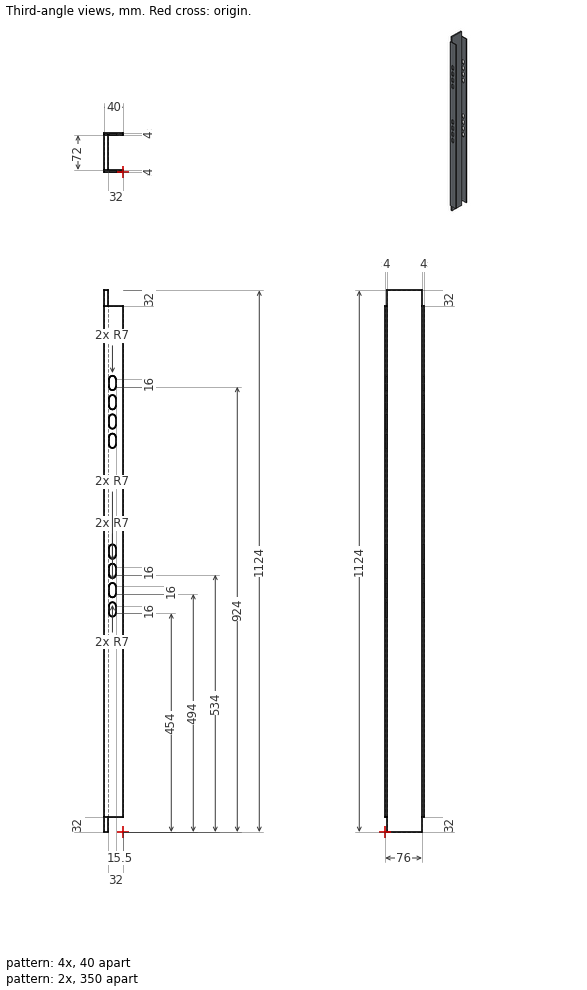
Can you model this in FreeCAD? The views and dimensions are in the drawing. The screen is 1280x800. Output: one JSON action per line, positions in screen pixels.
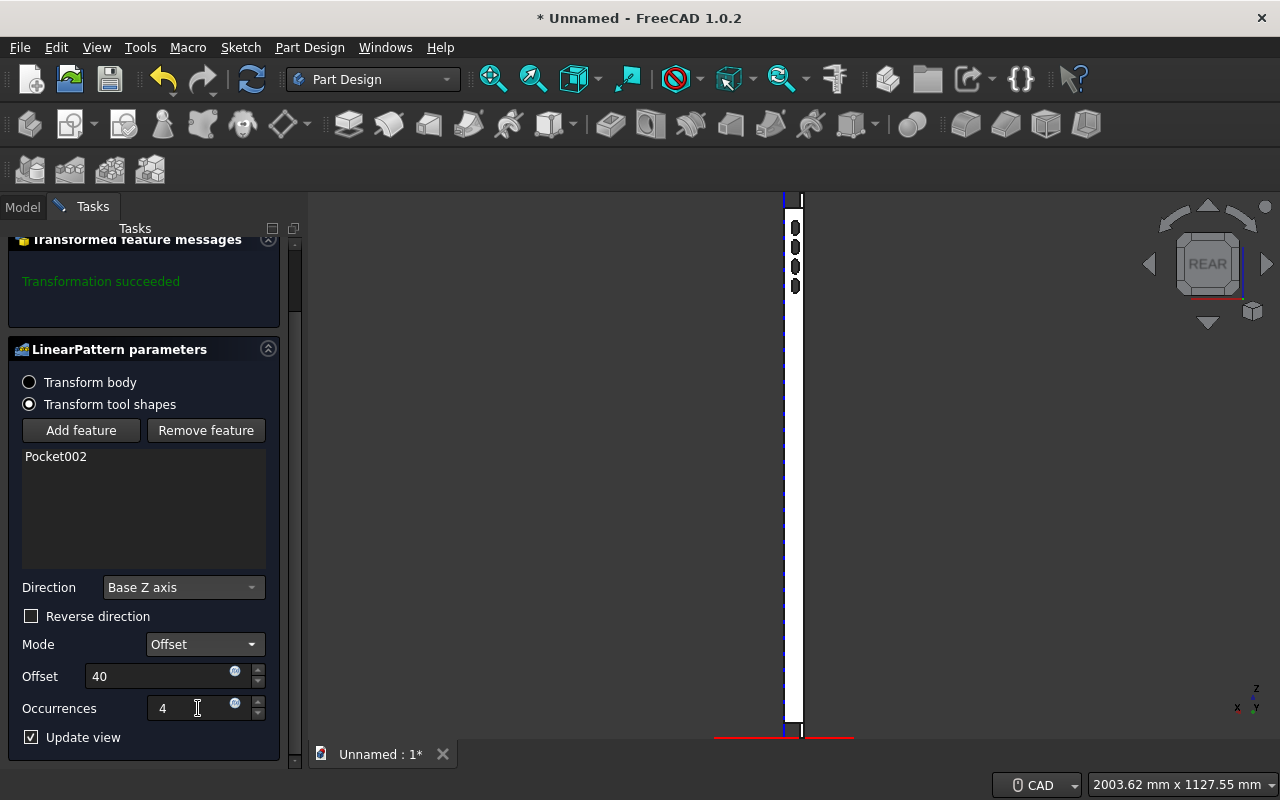
{"action": "left_click", "coordinate": [30, 616]}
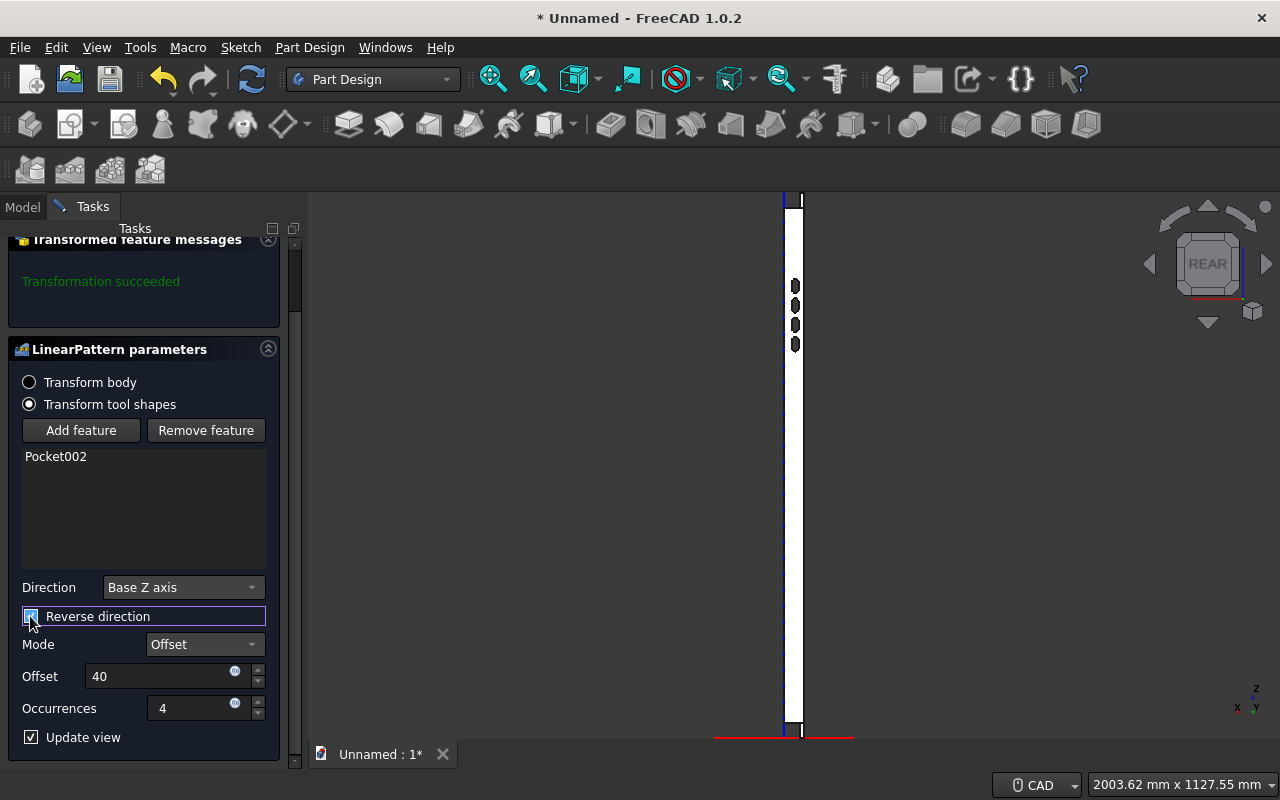
{"action": "scroll", "coordinate": [295, 503], "scroll_direction": "up", "scroll_amount": 2}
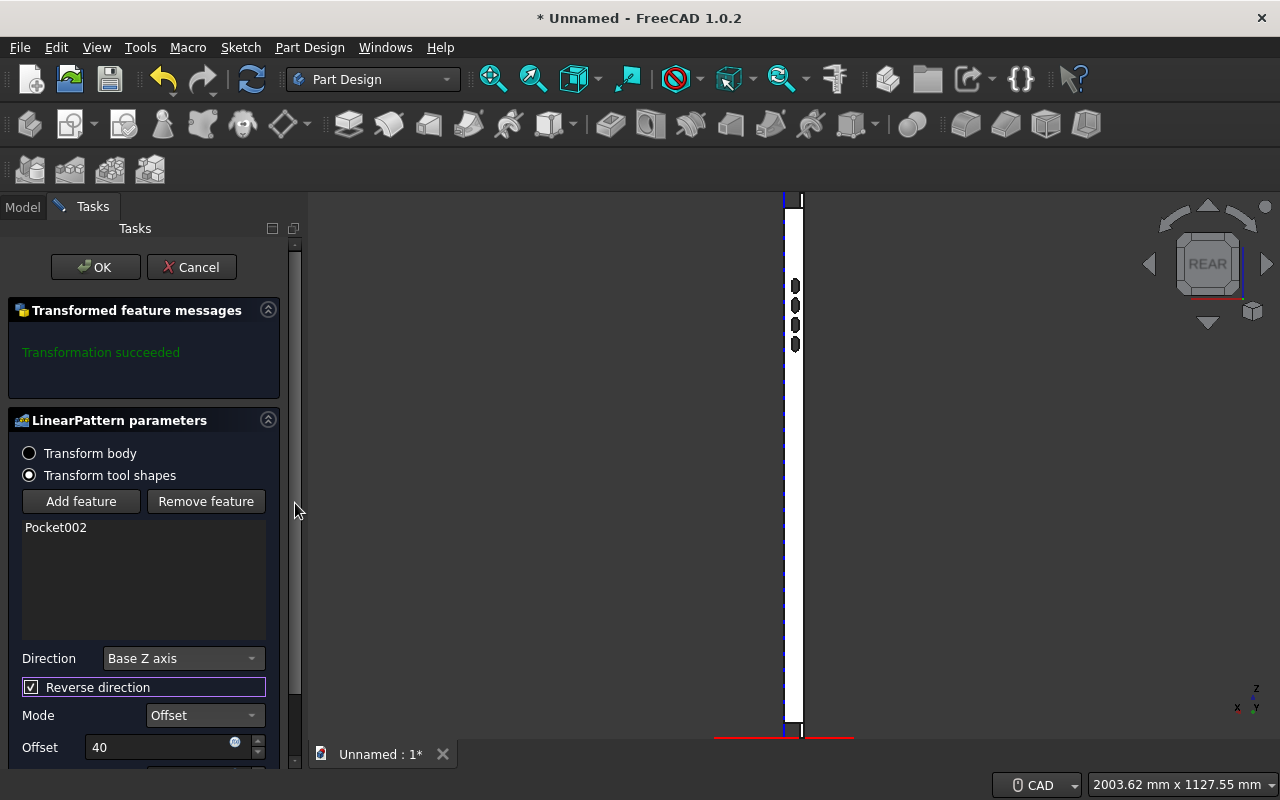
{"action": "left_click", "coordinate": [96, 267]}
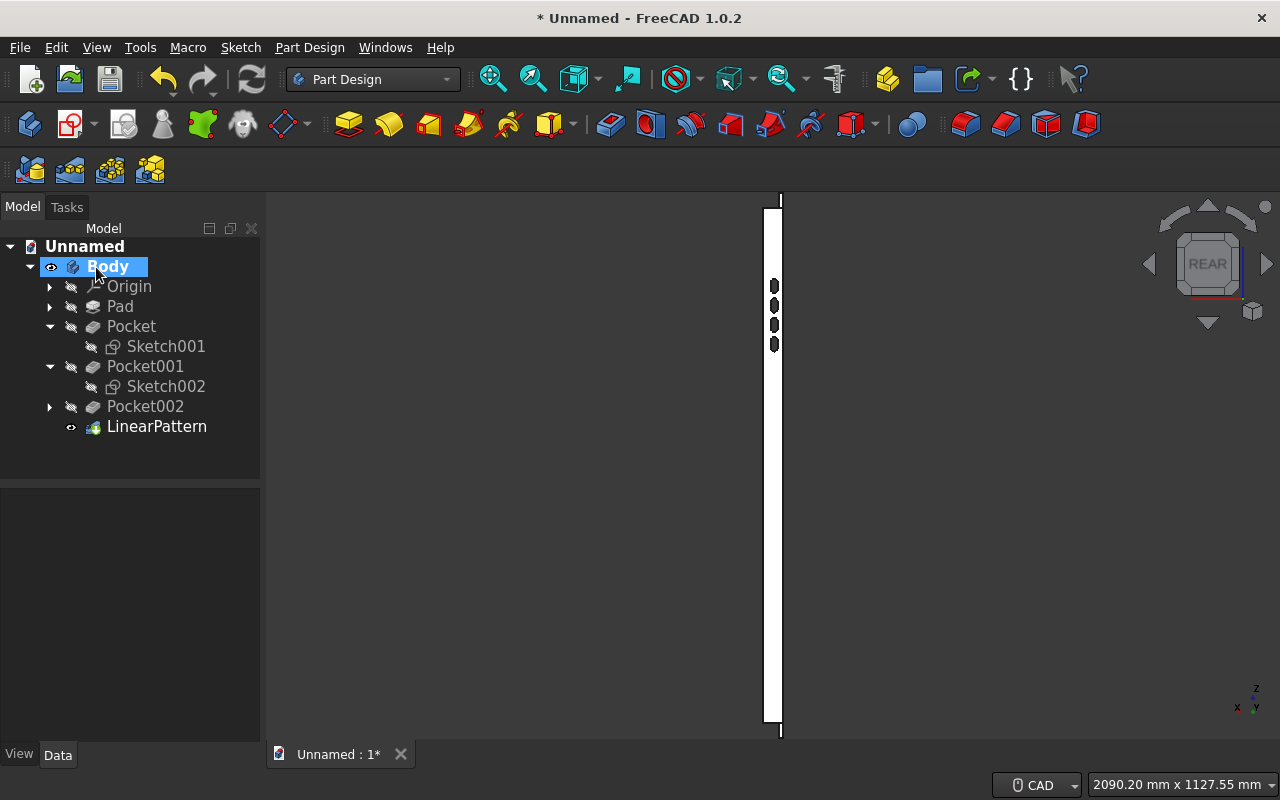
{"action": "left_click", "coordinate": [116, 407]}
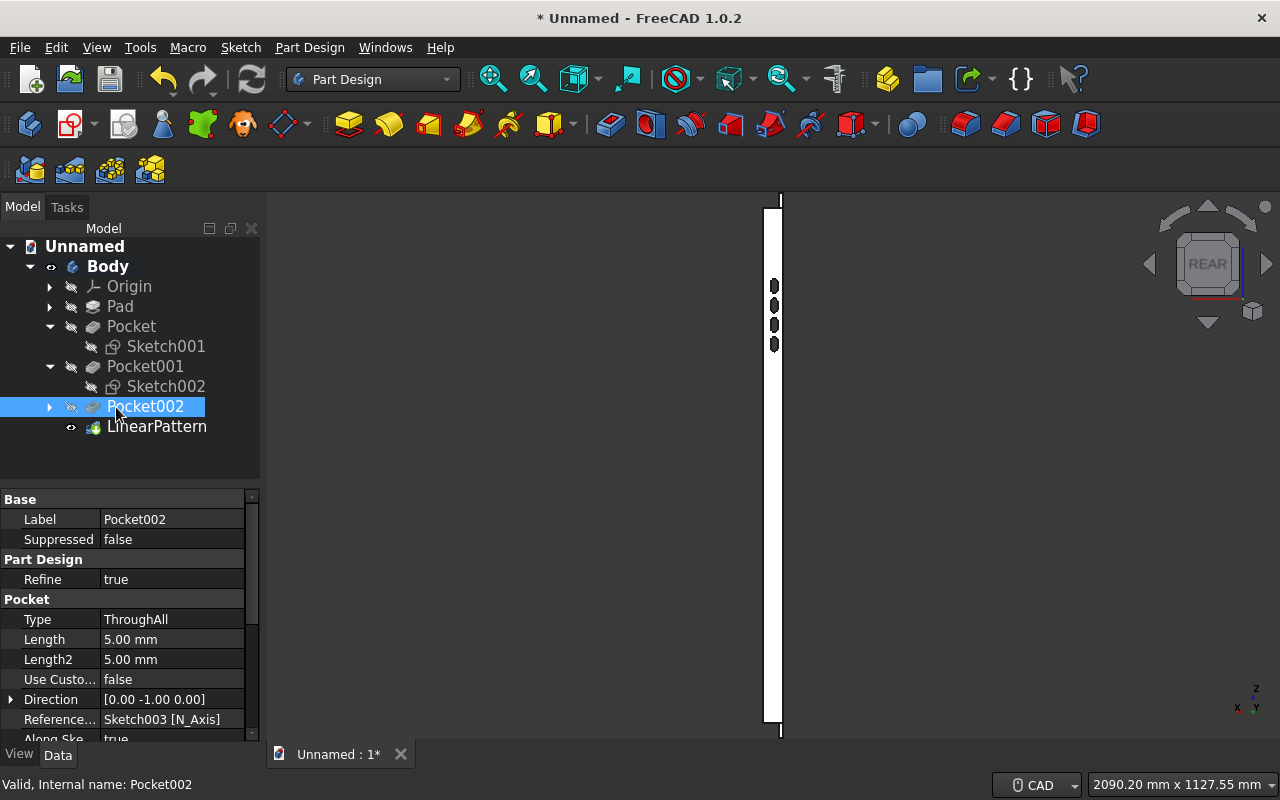
{"action": "left_click", "coordinate": [70, 170]}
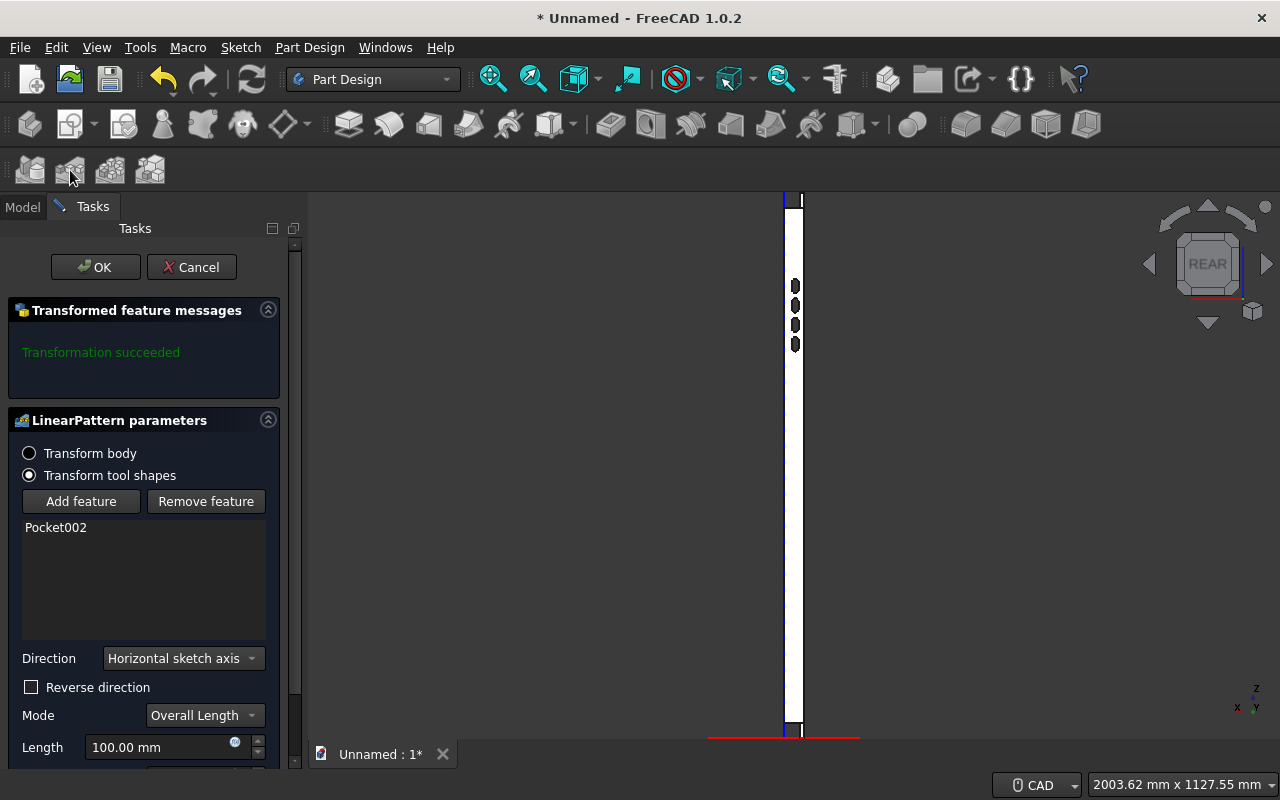
{"action": "left_click", "coordinate": [184, 658]}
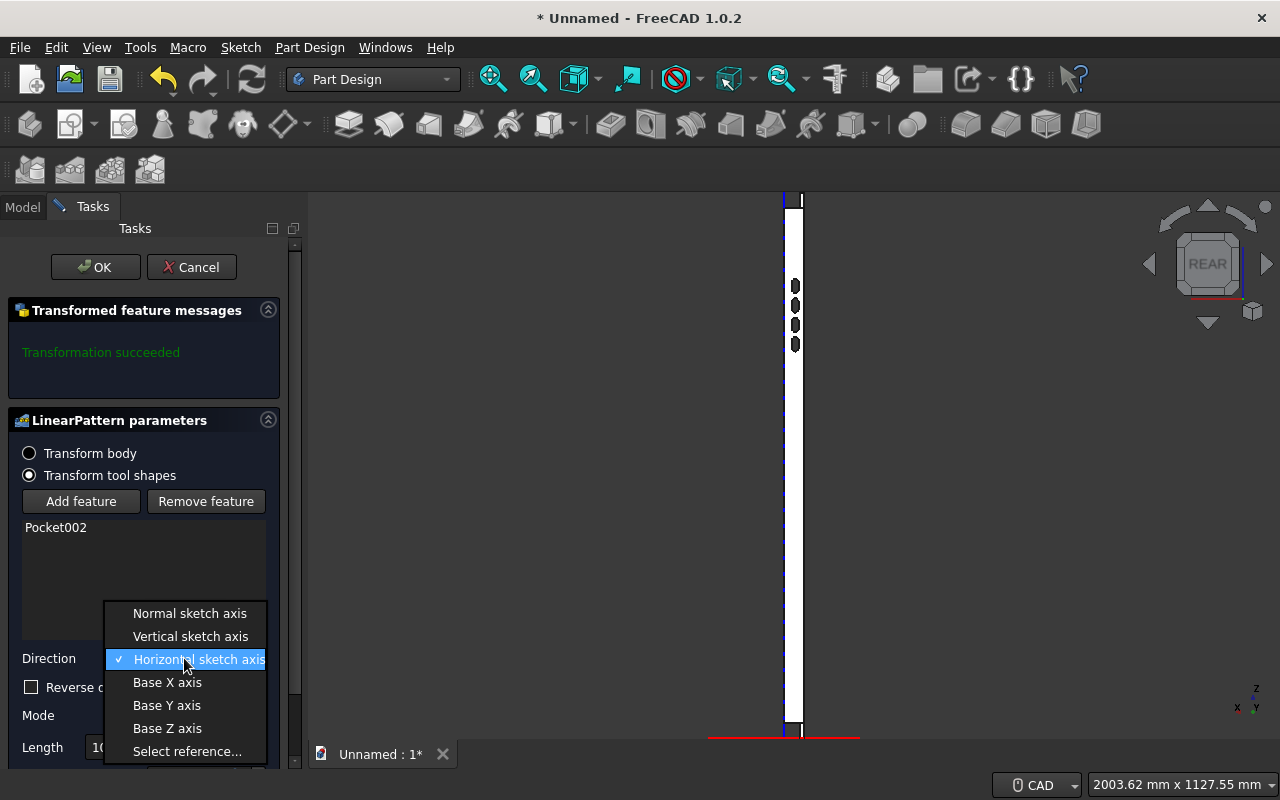
{"action": "left_click", "coordinate": [184, 728]}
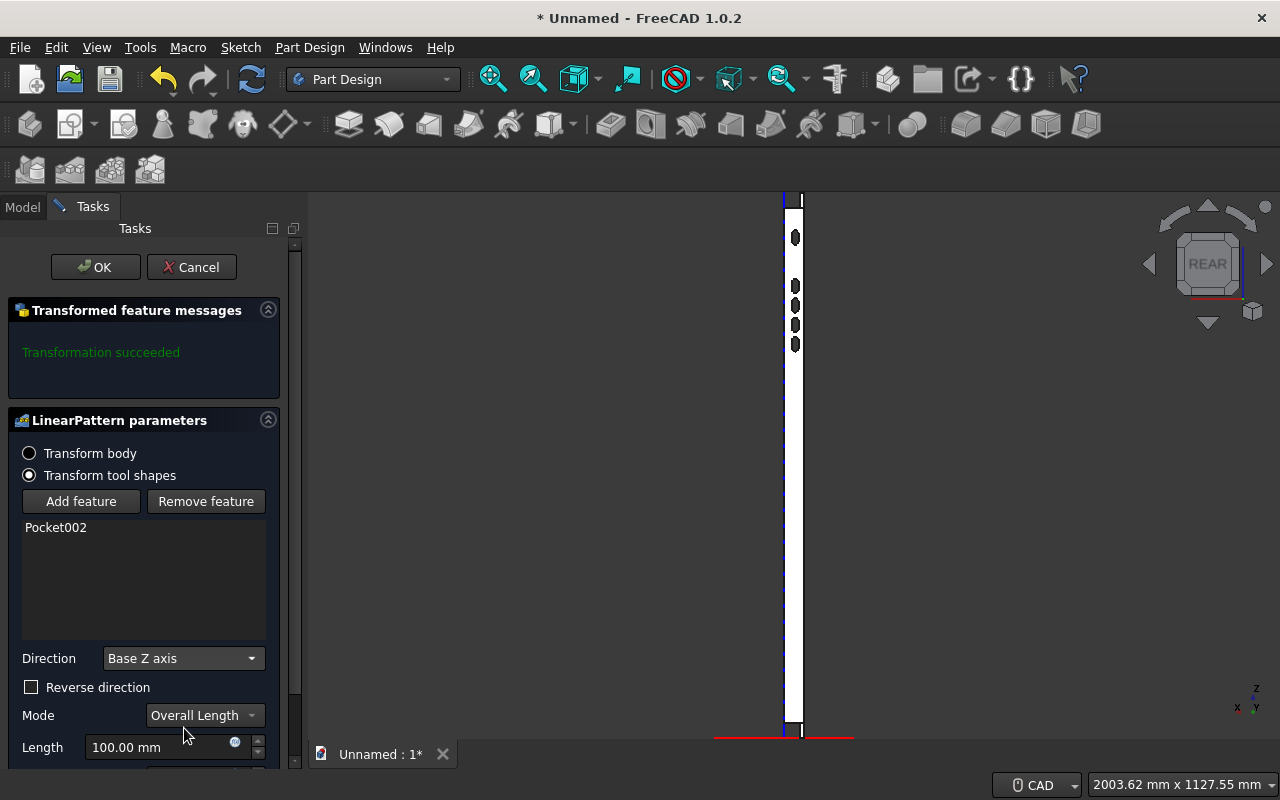
{"action": "left_click", "coordinate": [206, 716]}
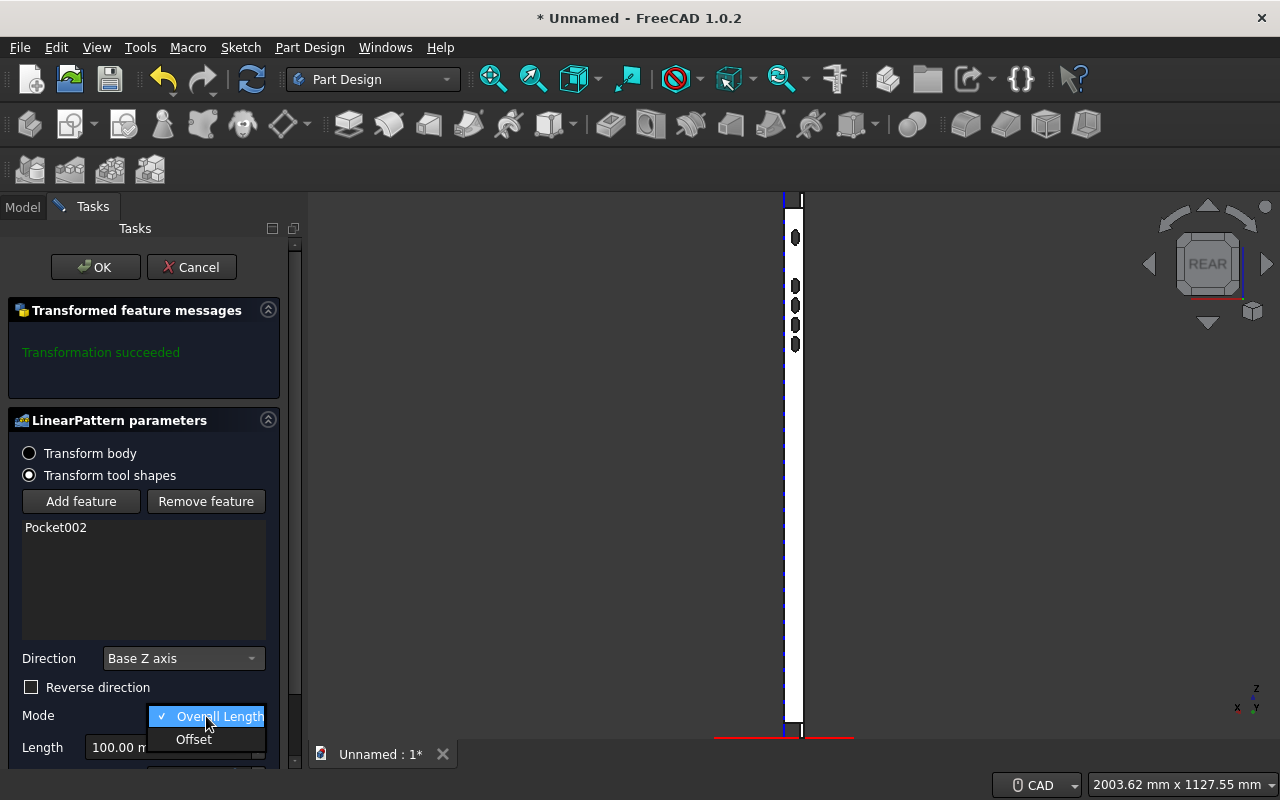
{"action": "left_click", "coordinate": [206, 740]}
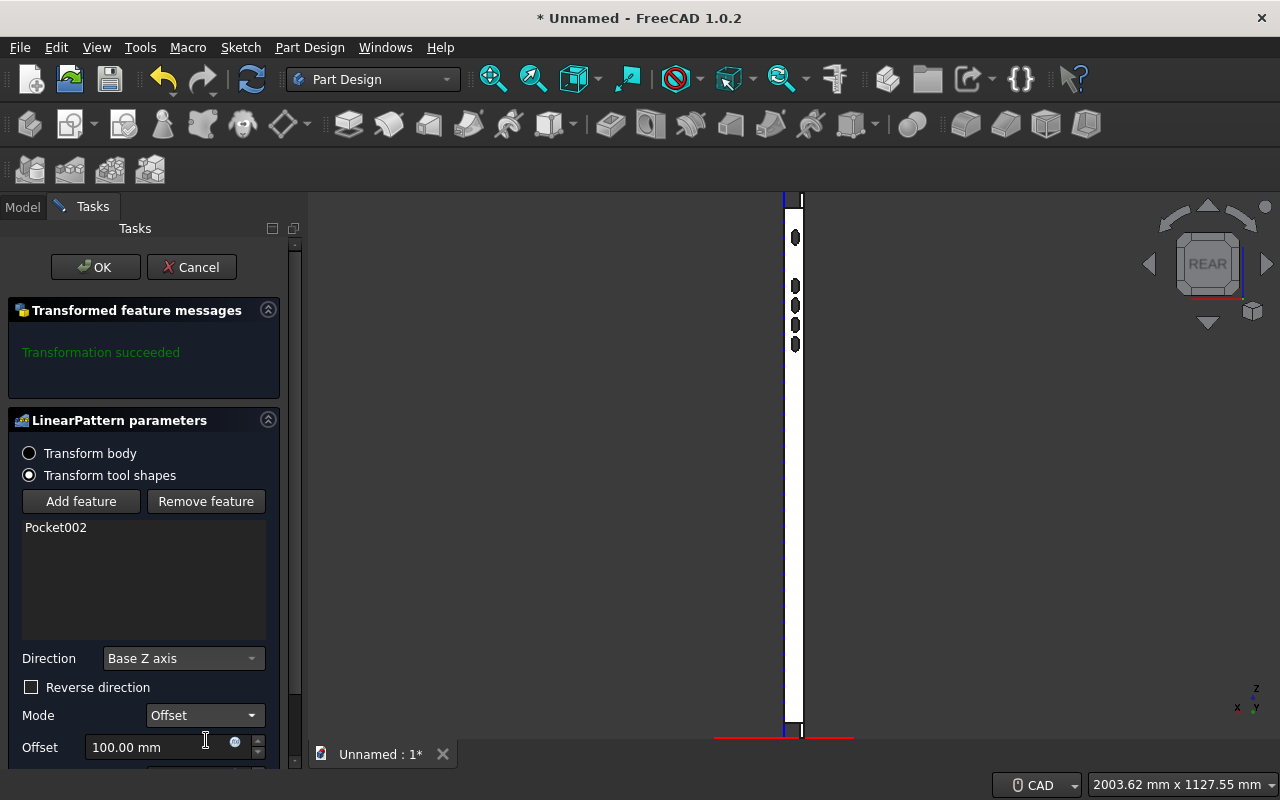
{"action": "triple_click", "coordinate": [168, 747]}